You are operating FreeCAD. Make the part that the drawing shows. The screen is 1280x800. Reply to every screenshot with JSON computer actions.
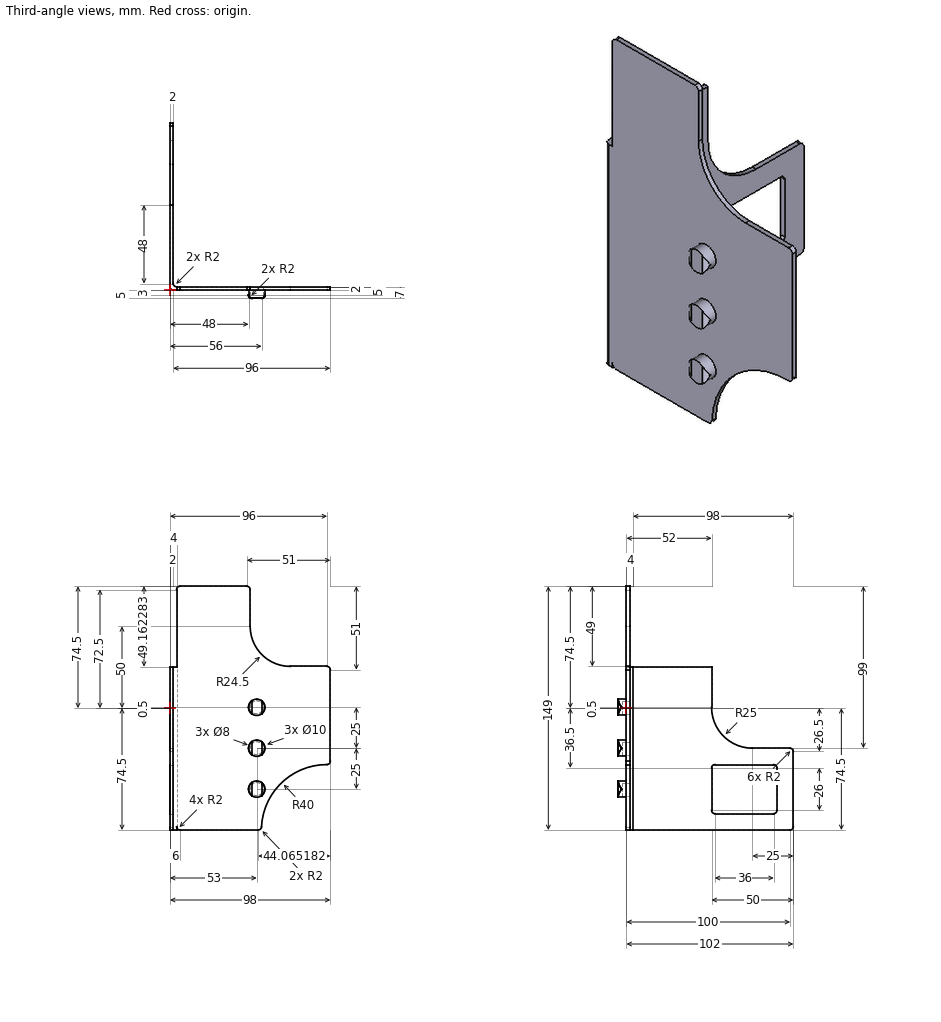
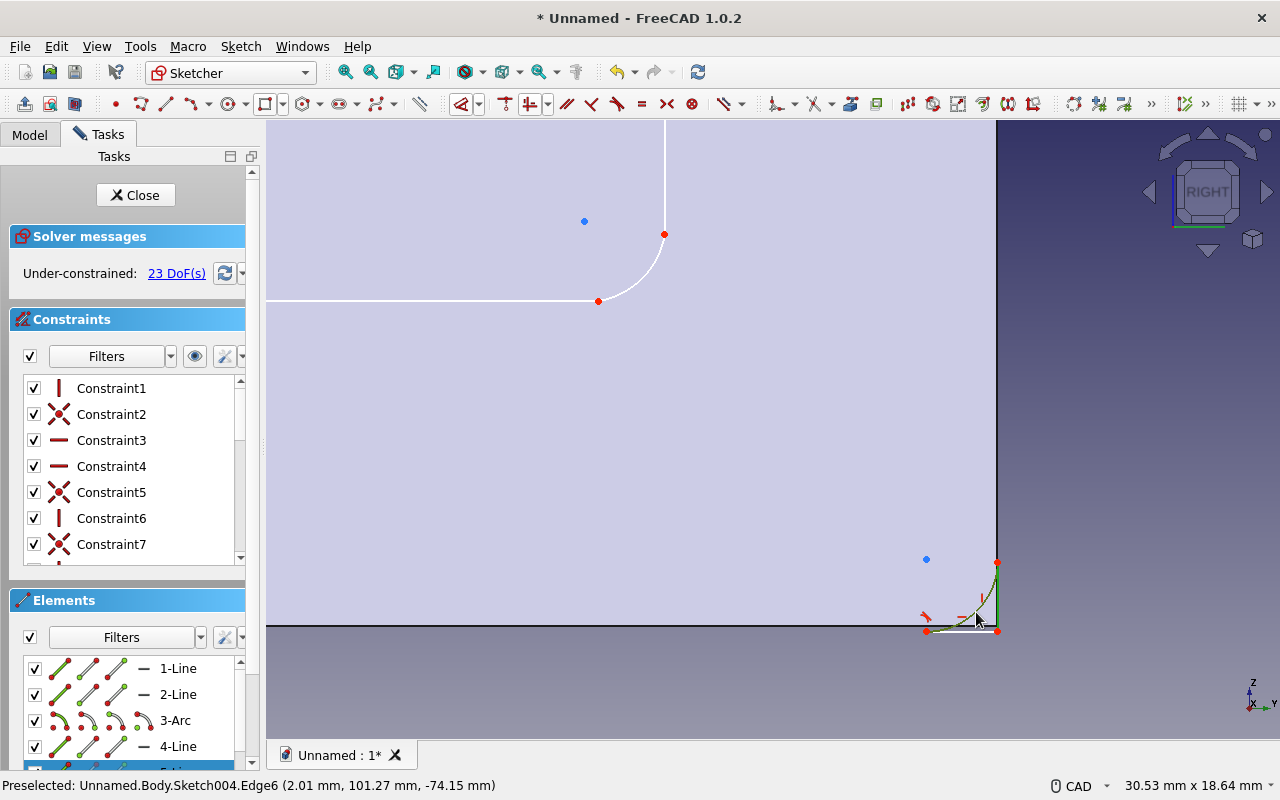
{"action": "key", "text": "t"}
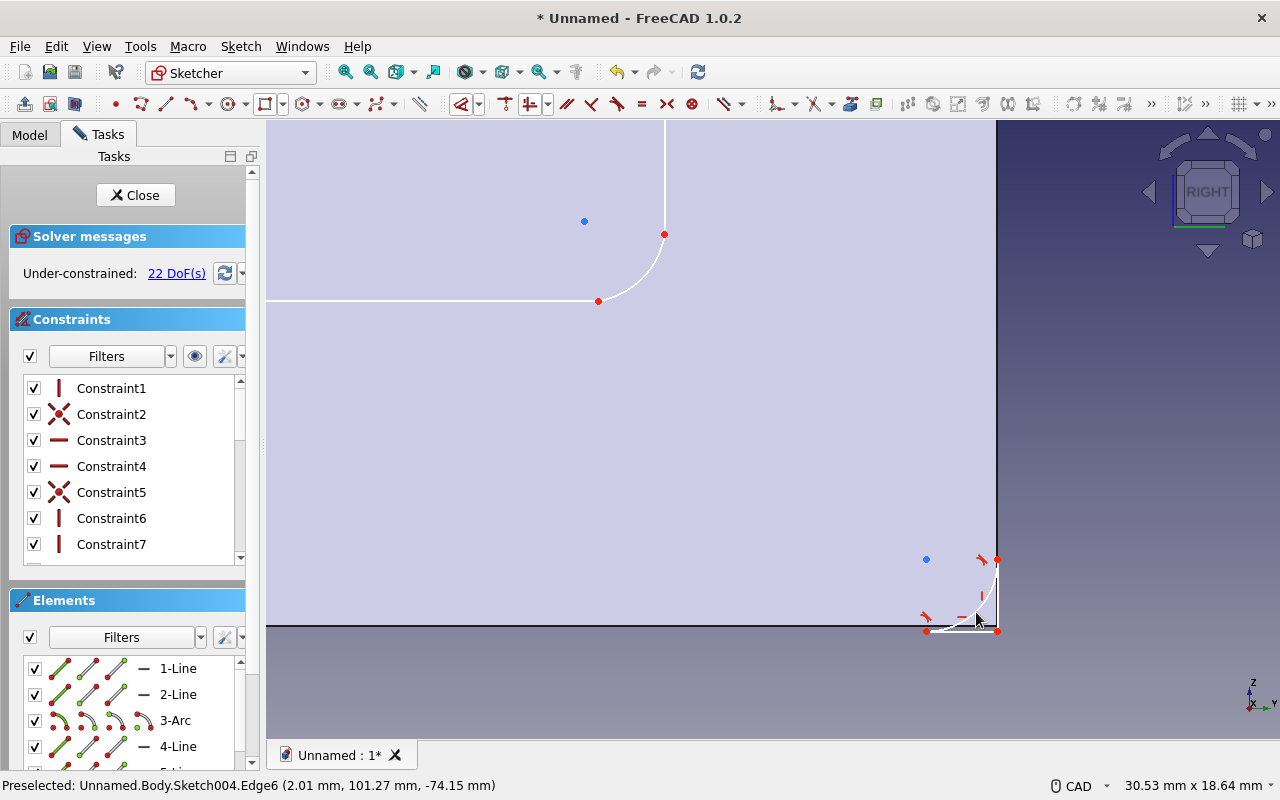
{"action": "scroll", "coordinate": [982, 636], "scroll_direction": "down", "scroll_amount": 9}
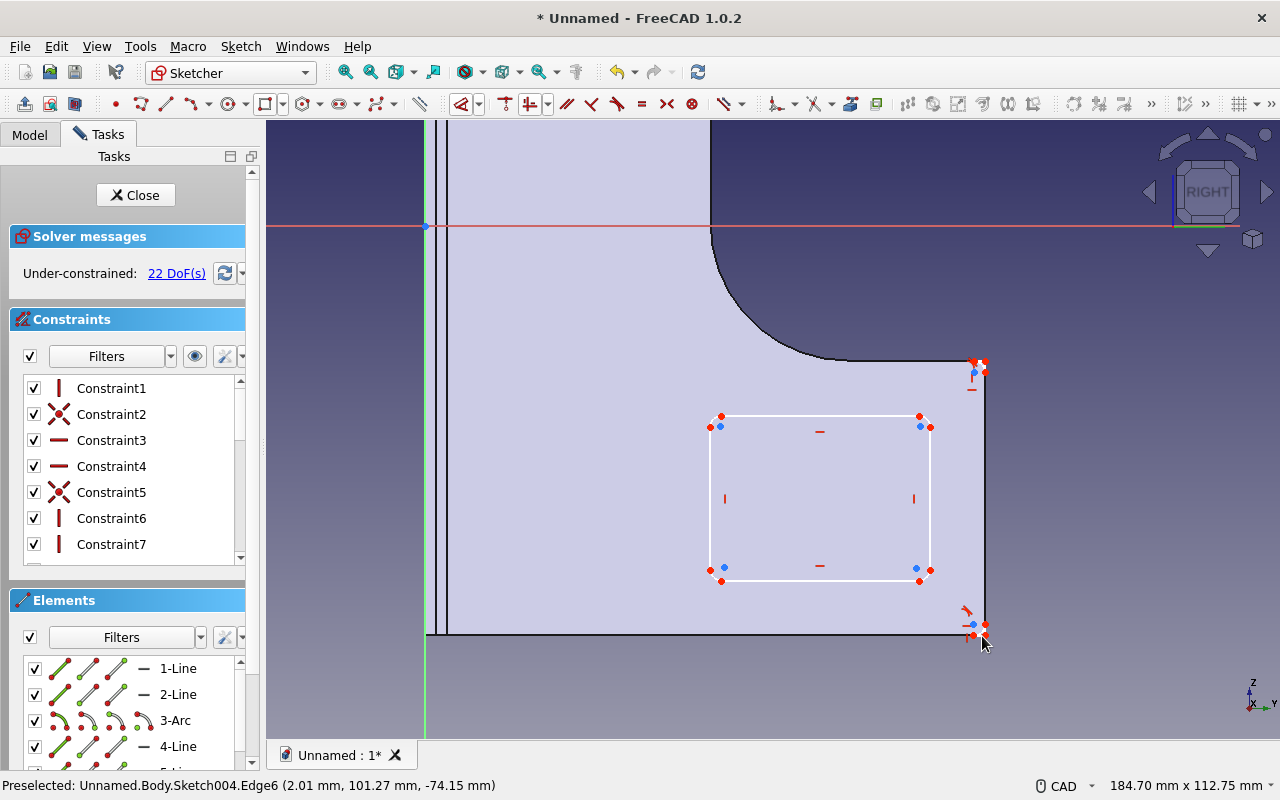
{"action": "left_click", "coordinate": [710, 470]}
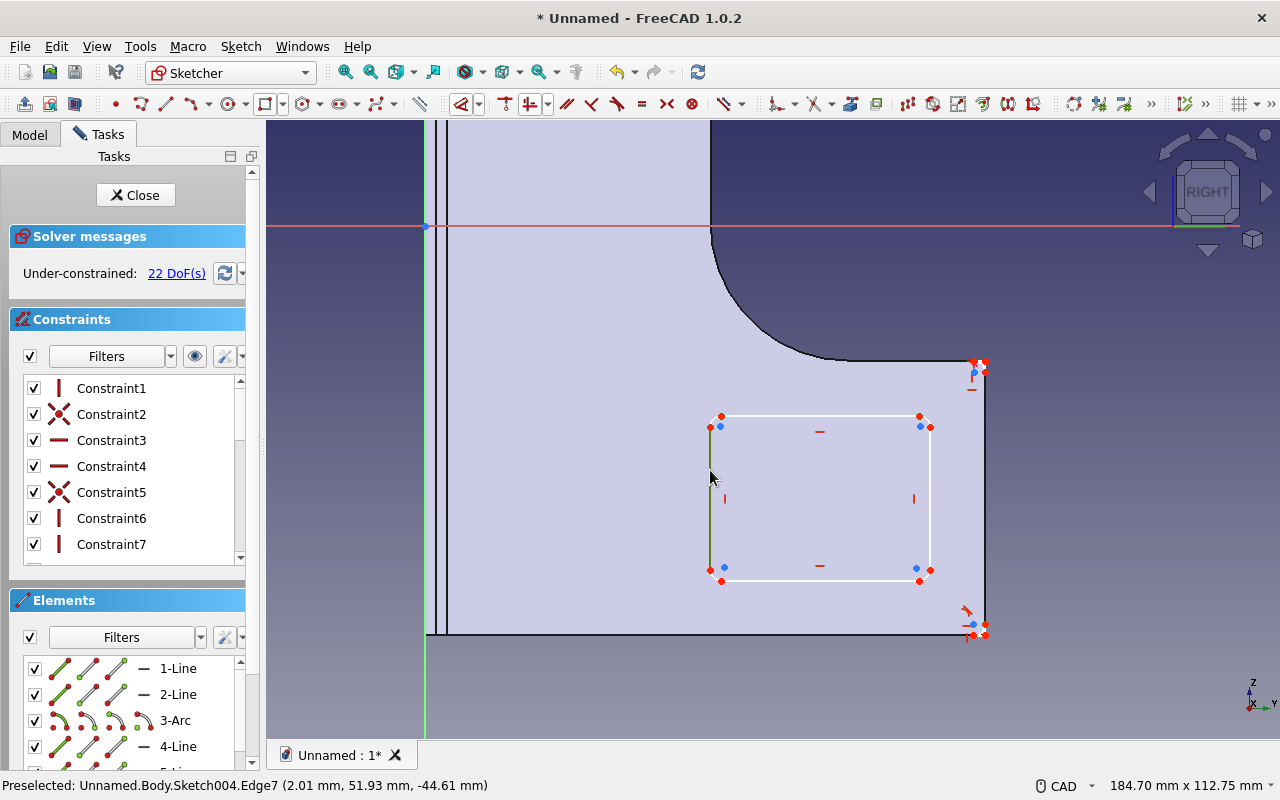
{"action": "scroll", "coordinate": [714, 577], "scroll_direction": "up", "scroll_amount": 3}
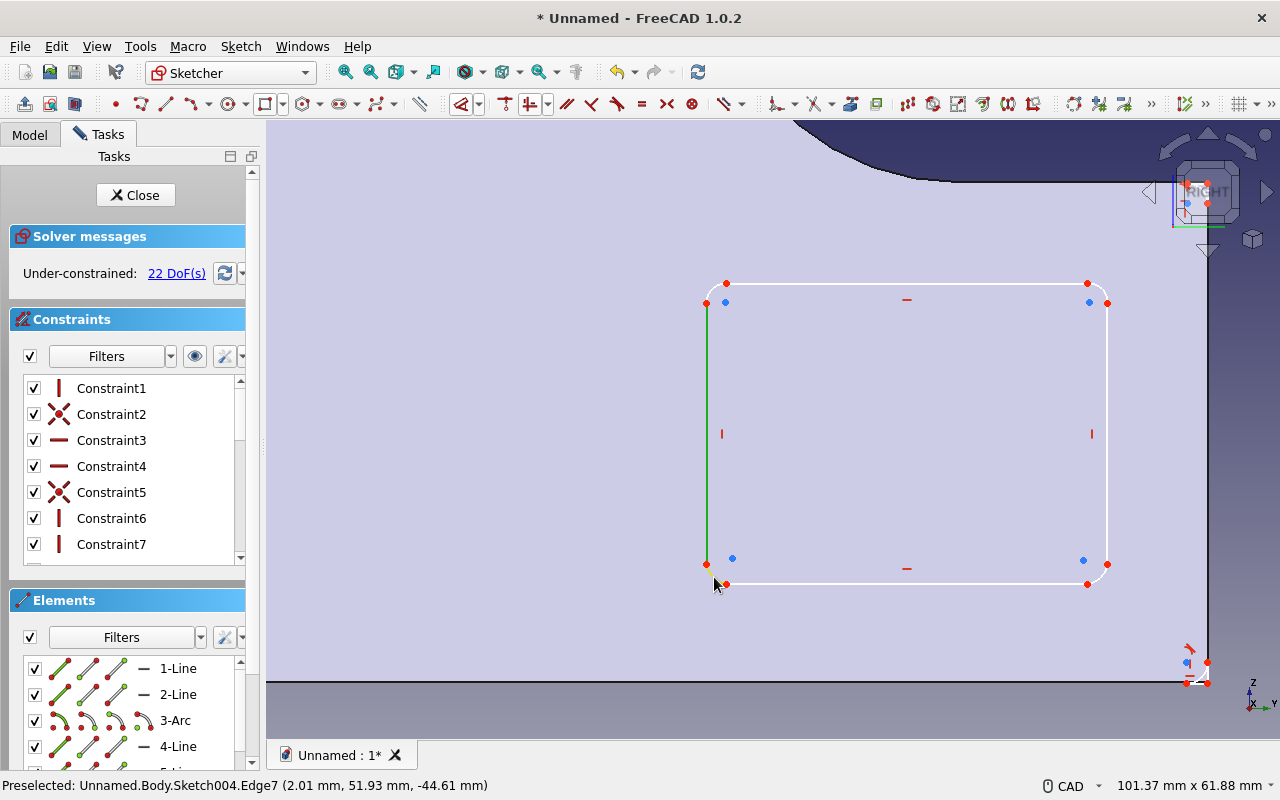
{"action": "left_click", "coordinate": [714, 577]}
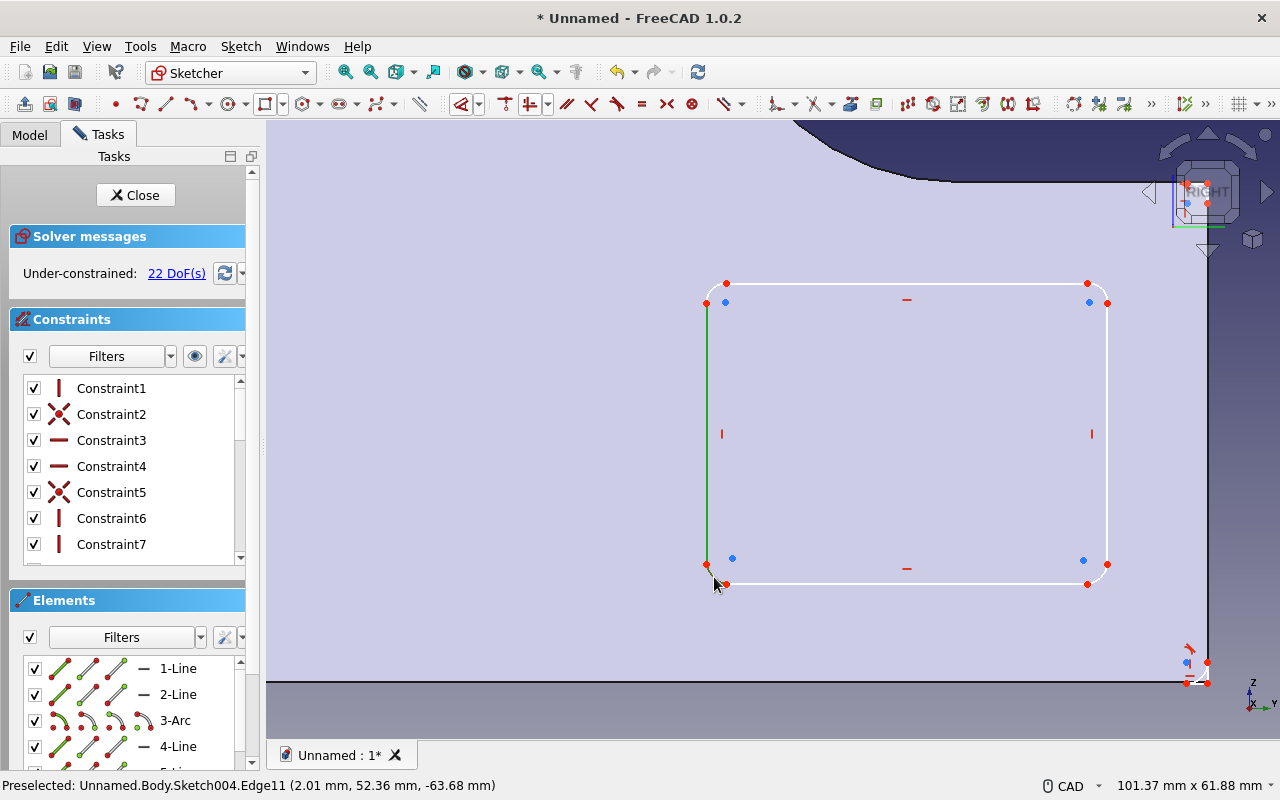
{"action": "key", "text": "t"}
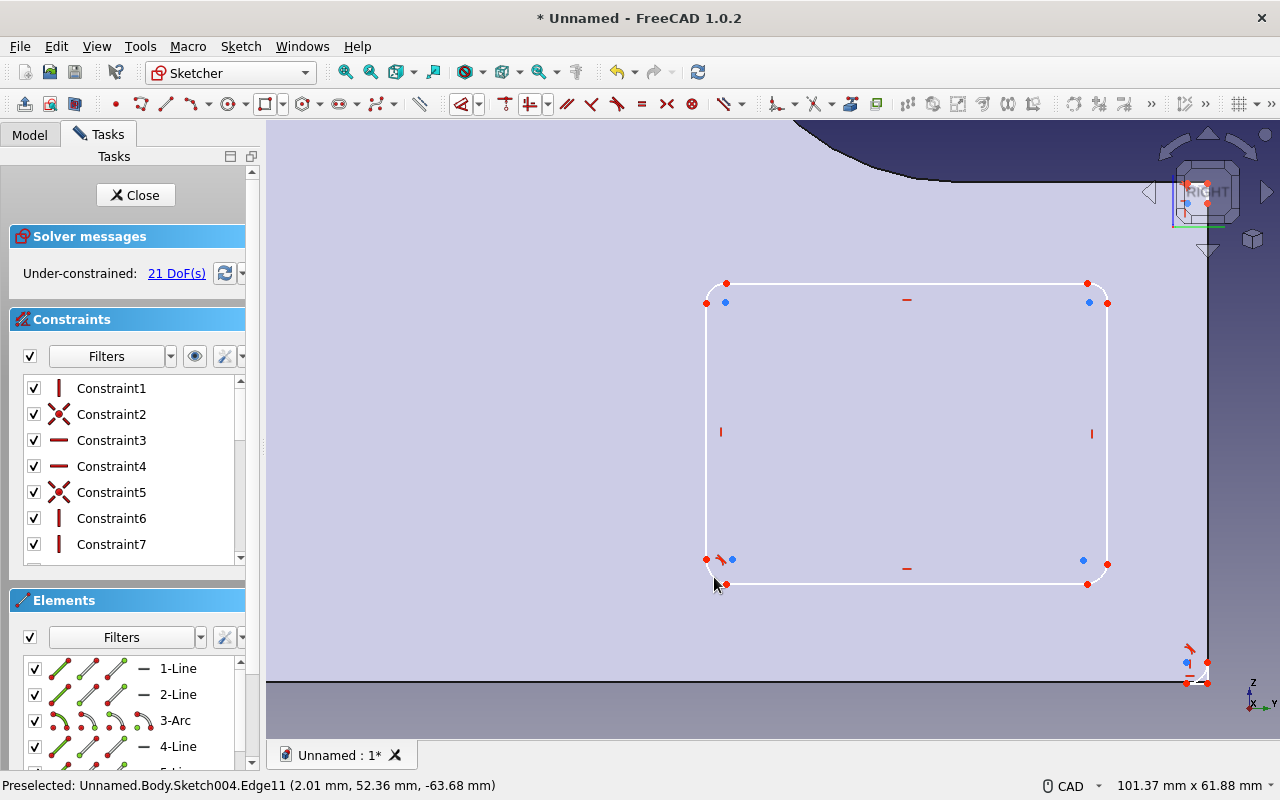
{"action": "left_click", "coordinate": [706, 380]}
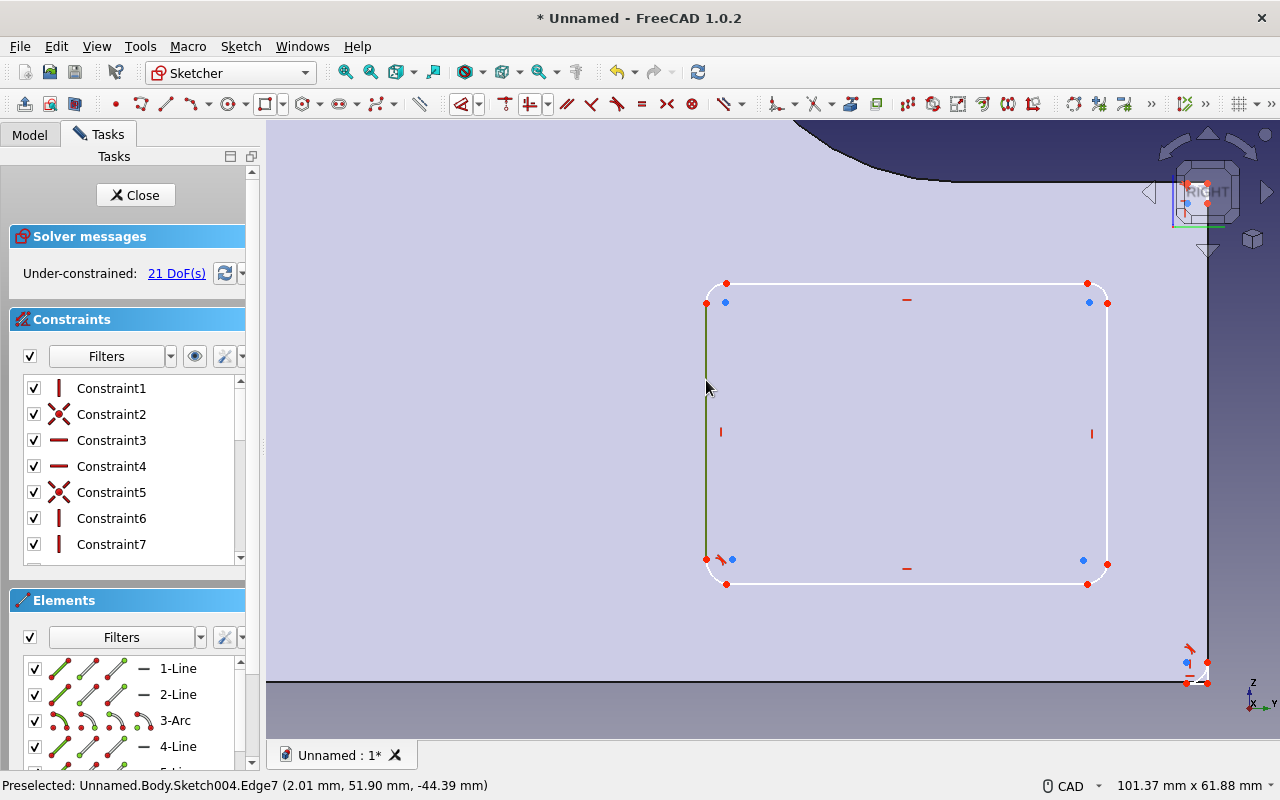
{"action": "scroll", "coordinate": [717, 285], "scroll_direction": "up", "scroll_amount": 2}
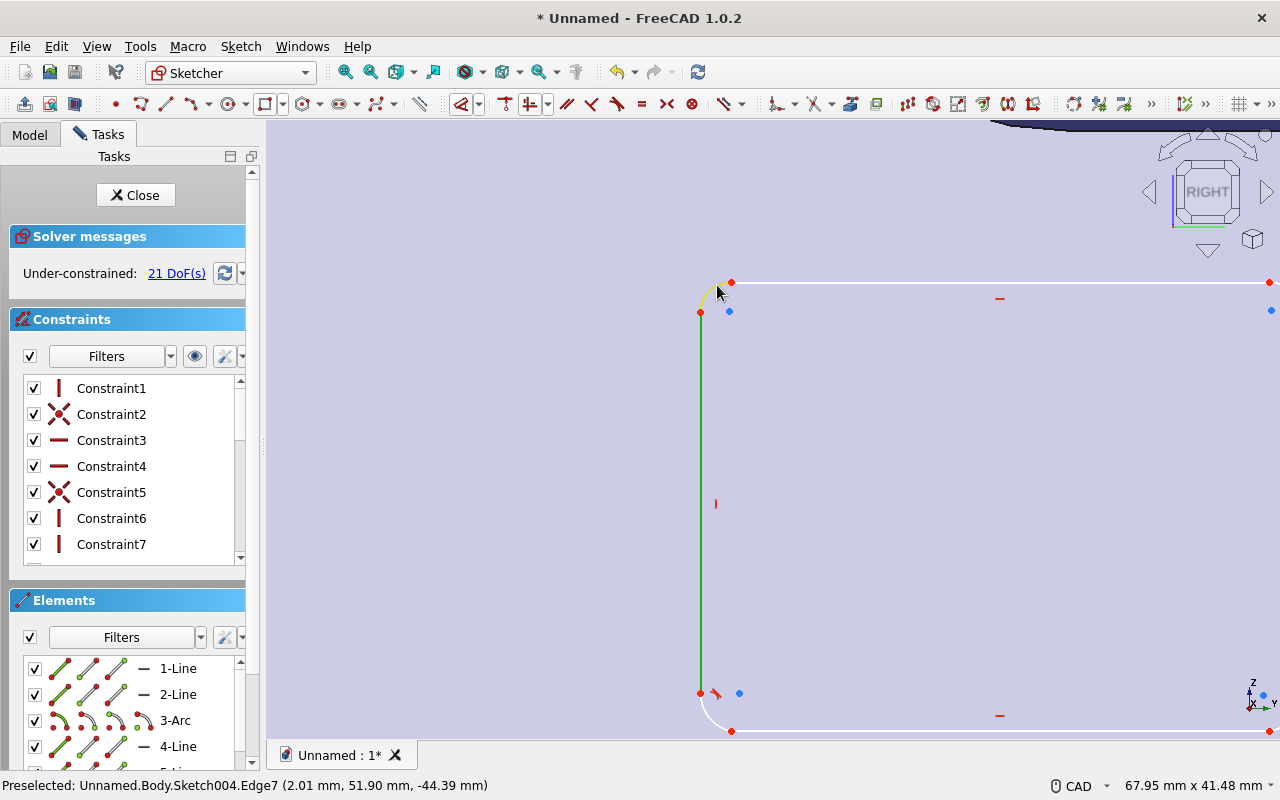
{"action": "left_click", "coordinate": [717, 286]}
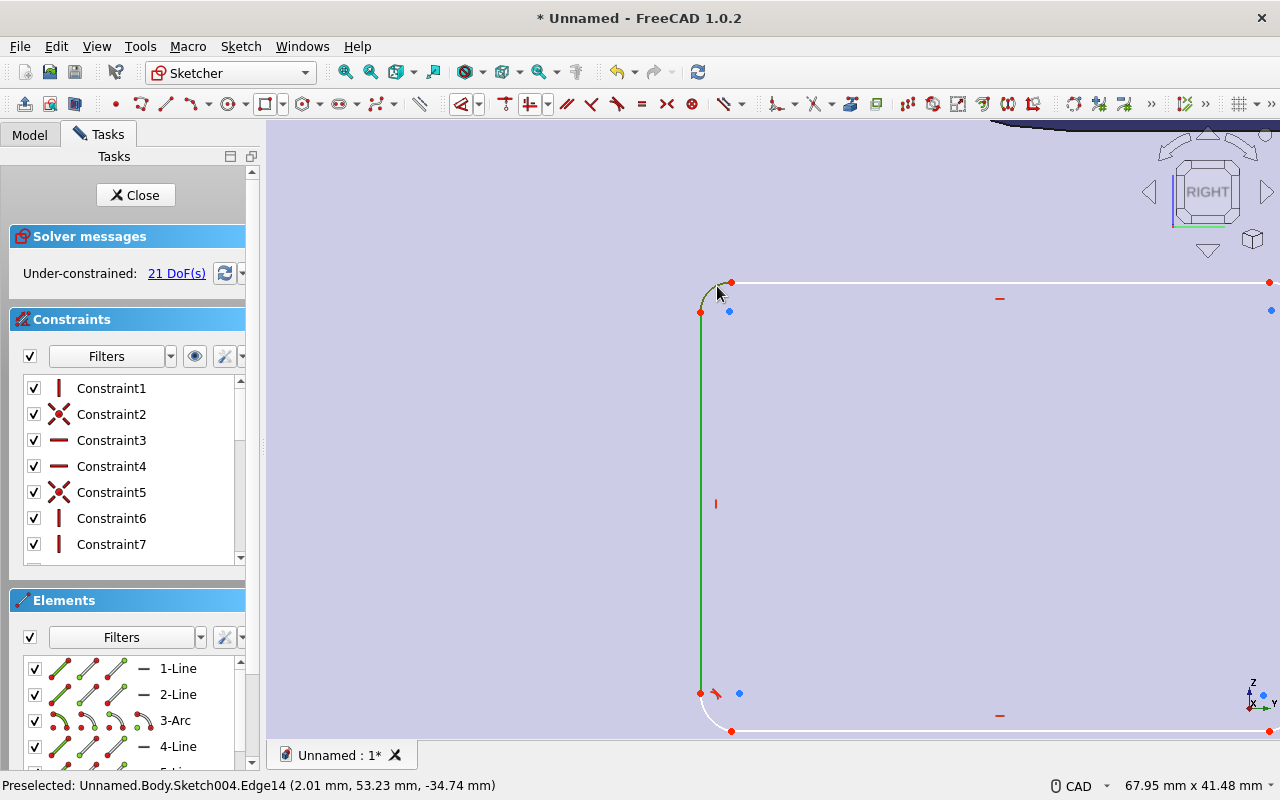
{"action": "key", "text": "t"}